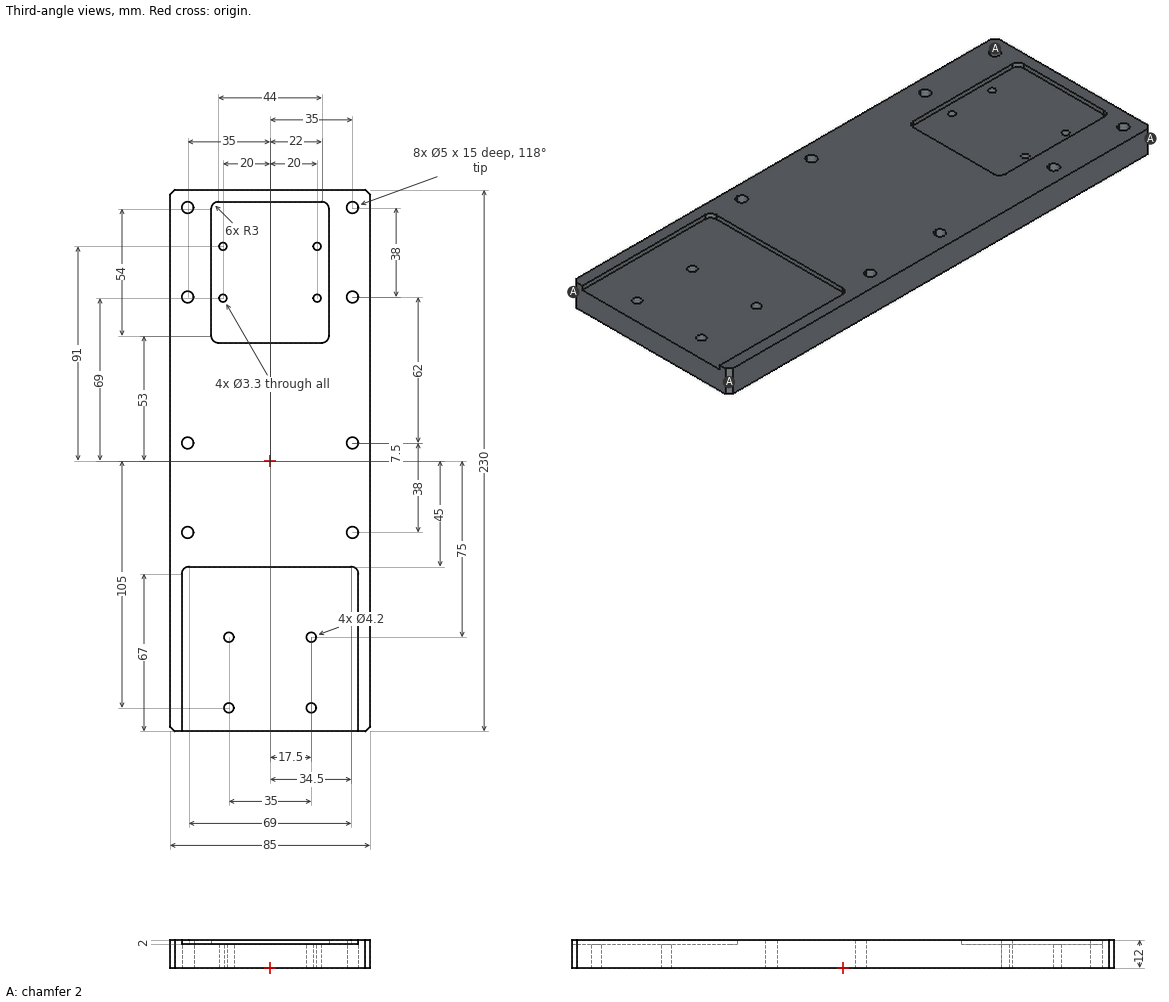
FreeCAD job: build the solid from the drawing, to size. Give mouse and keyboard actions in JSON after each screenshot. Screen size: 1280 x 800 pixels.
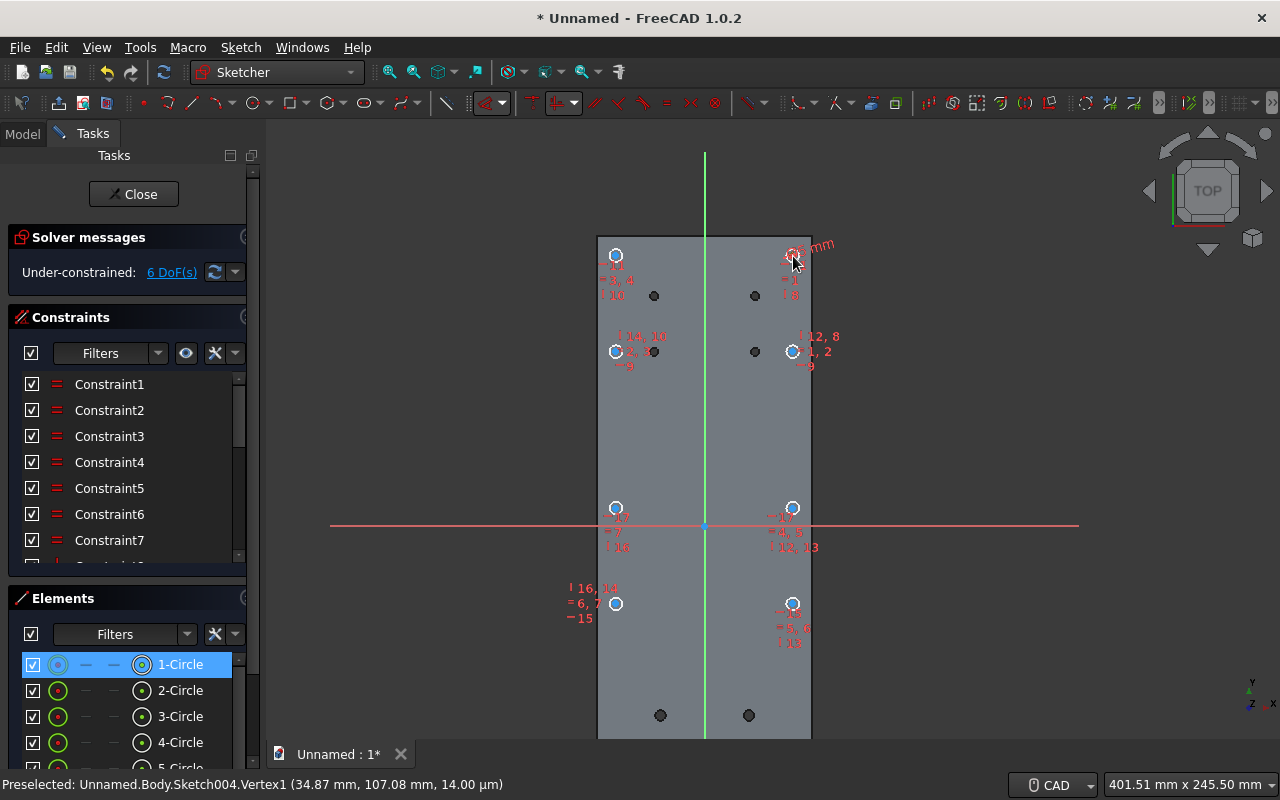
{"action": "left_click", "coordinate": [504, 104]}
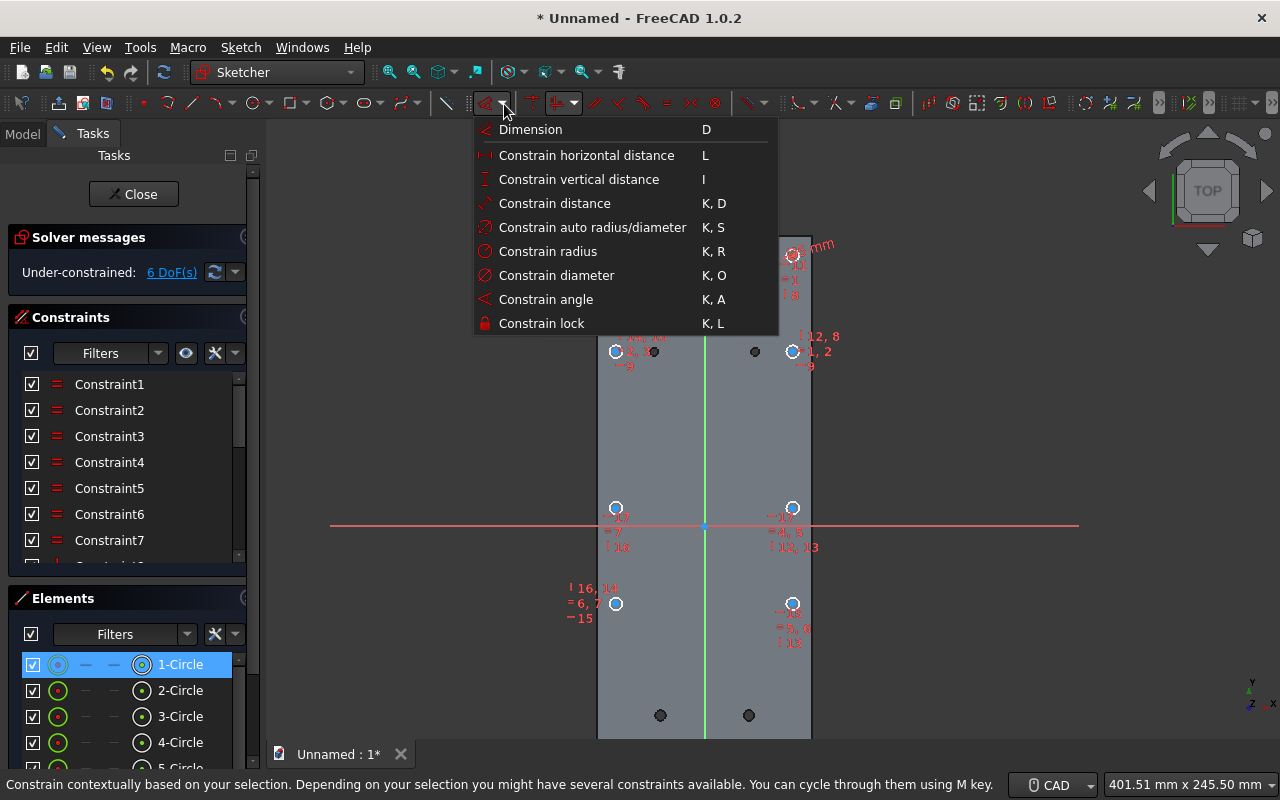
{"action": "left_click", "coordinate": [626, 155]}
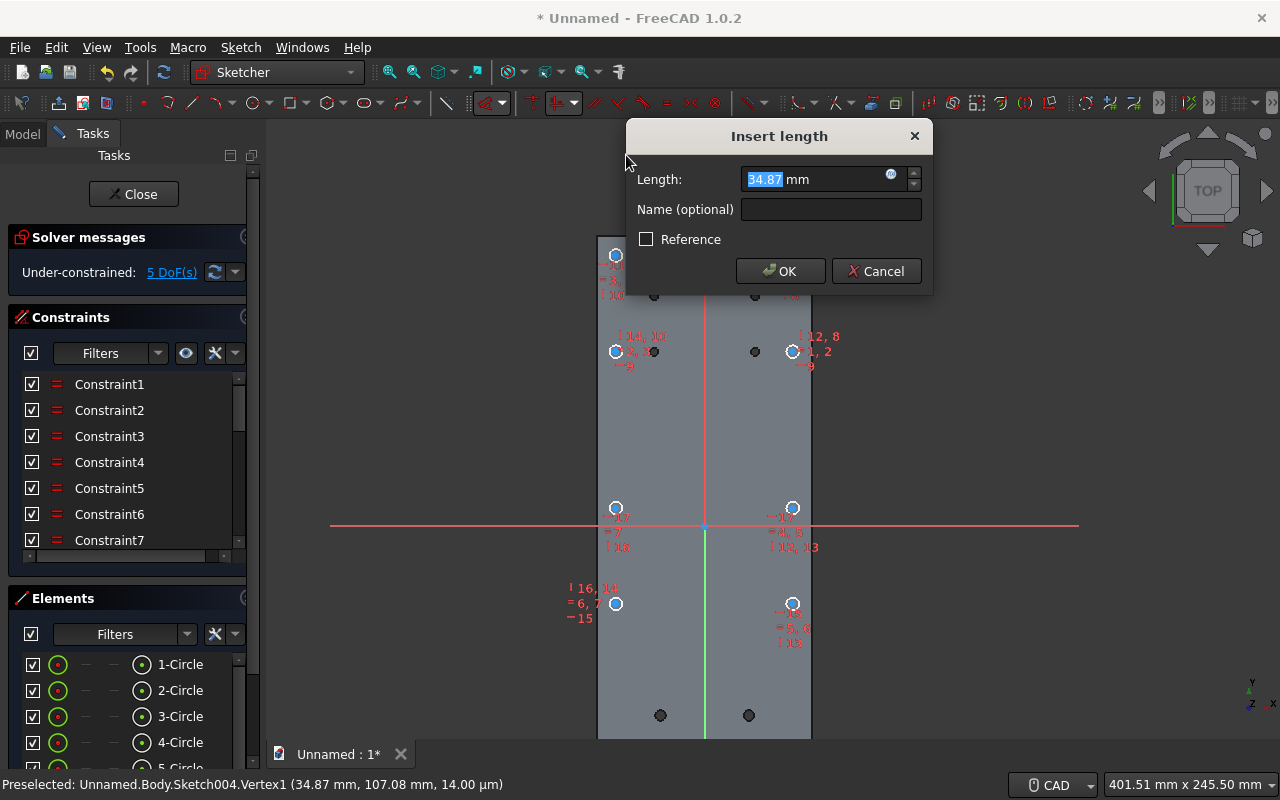
{"action": "type", "text": "35"}
{"action": "key", "text": "Return"}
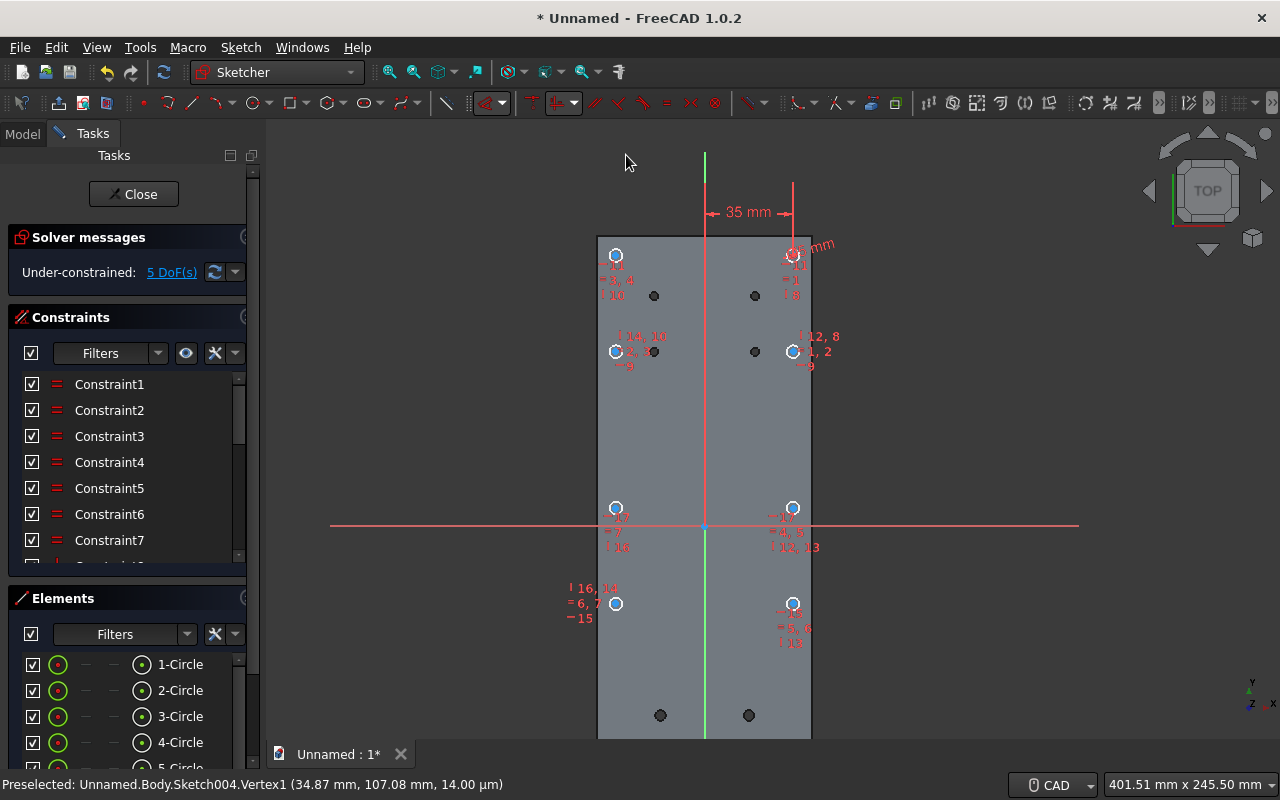
{"action": "left_click", "coordinate": [616, 352]}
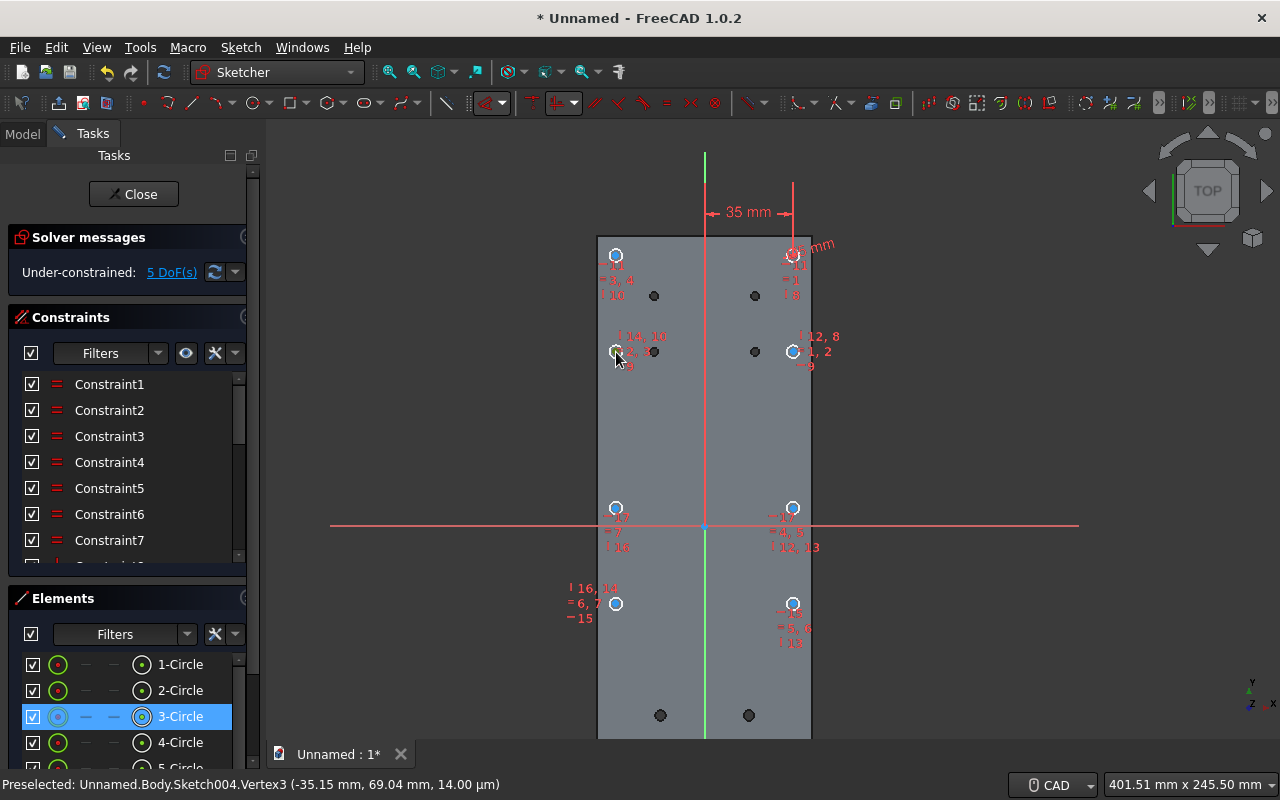
{"action": "key", "text": "l"}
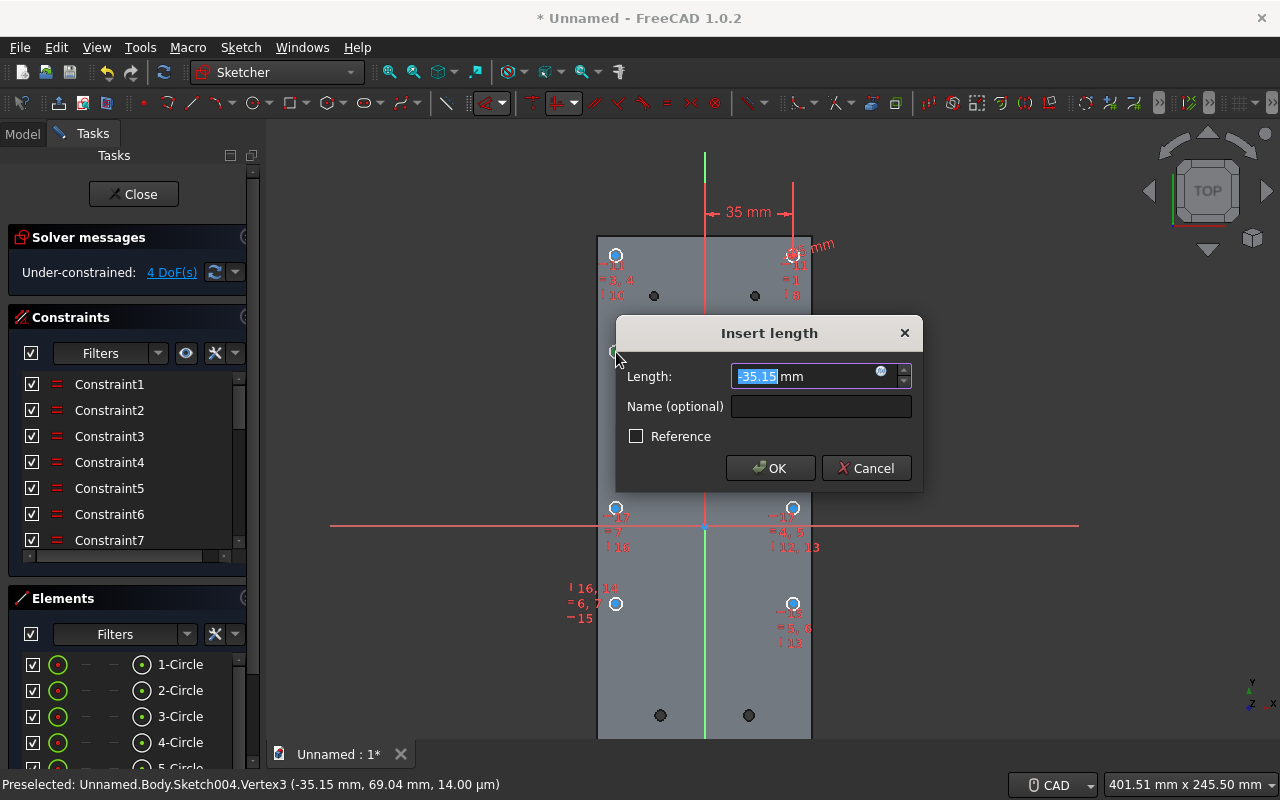
{"action": "type", "text": "-35"}
{"action": "key", "text": "Return"}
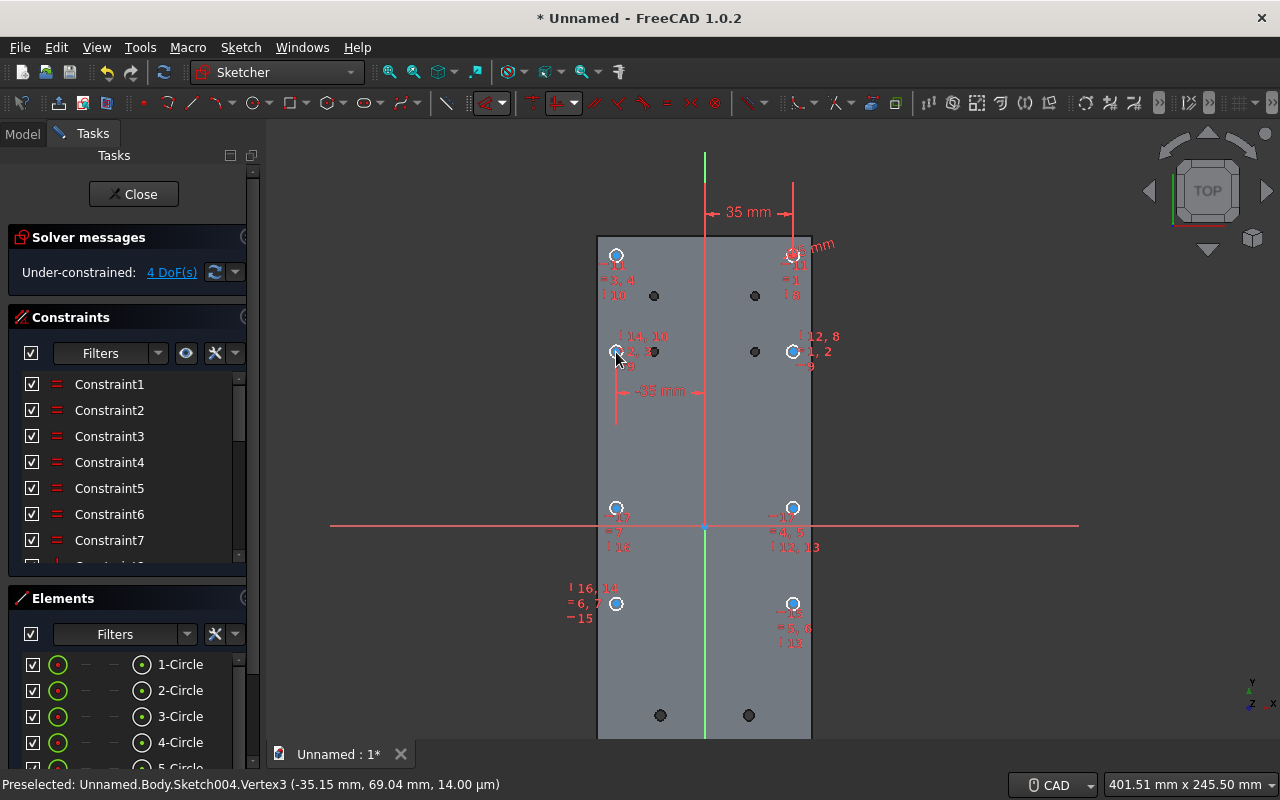
{"action": "scroll", "coordinate": [793, 508], "scroll_direction": "up", "scroll_amount": 4}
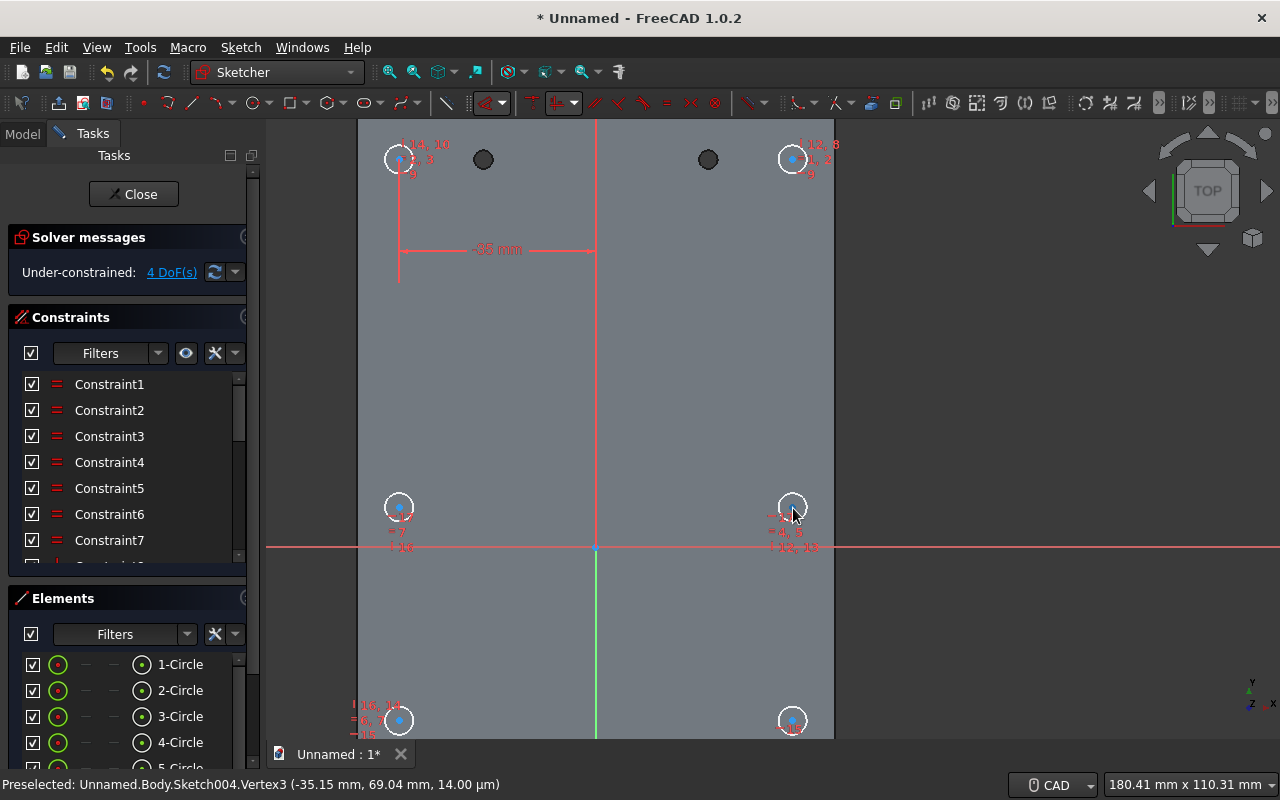
{"action": "left_click", "coordinate": [793, 507]}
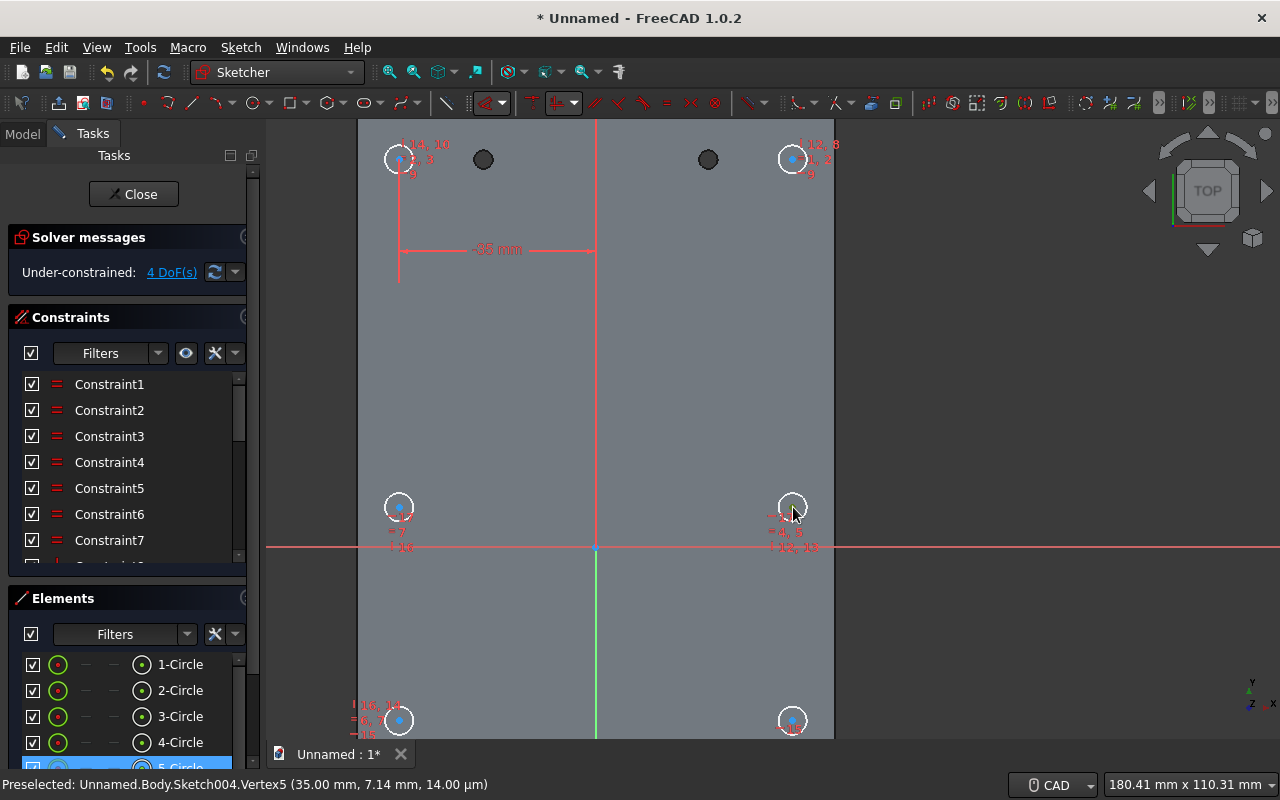
{"action": "key", "text": "i"}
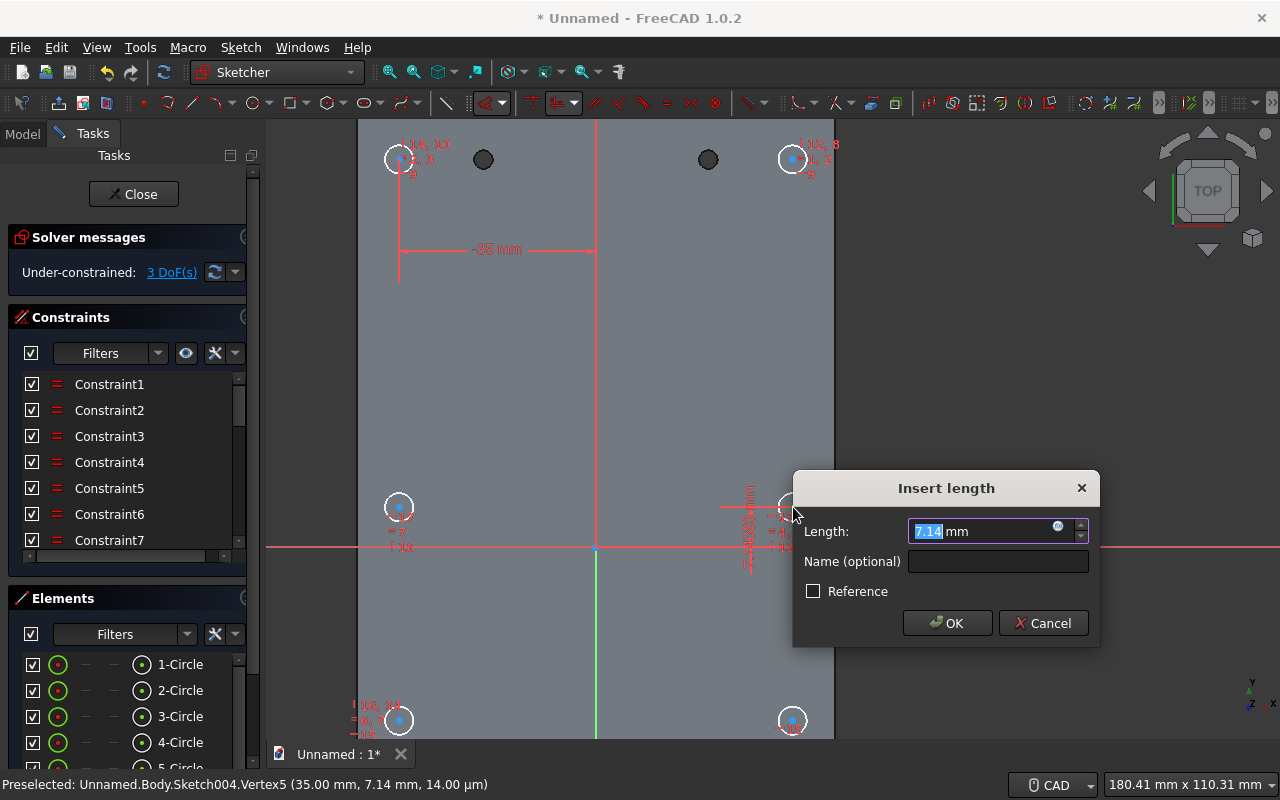
{"action": "type", "text": "7.5"}
{"action": "key", "text": "Return"}